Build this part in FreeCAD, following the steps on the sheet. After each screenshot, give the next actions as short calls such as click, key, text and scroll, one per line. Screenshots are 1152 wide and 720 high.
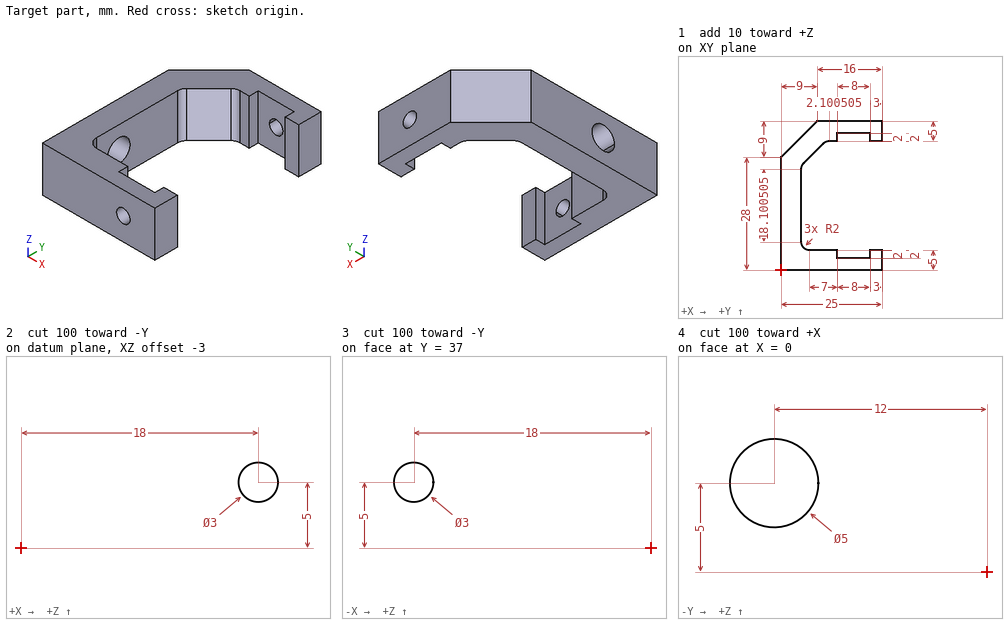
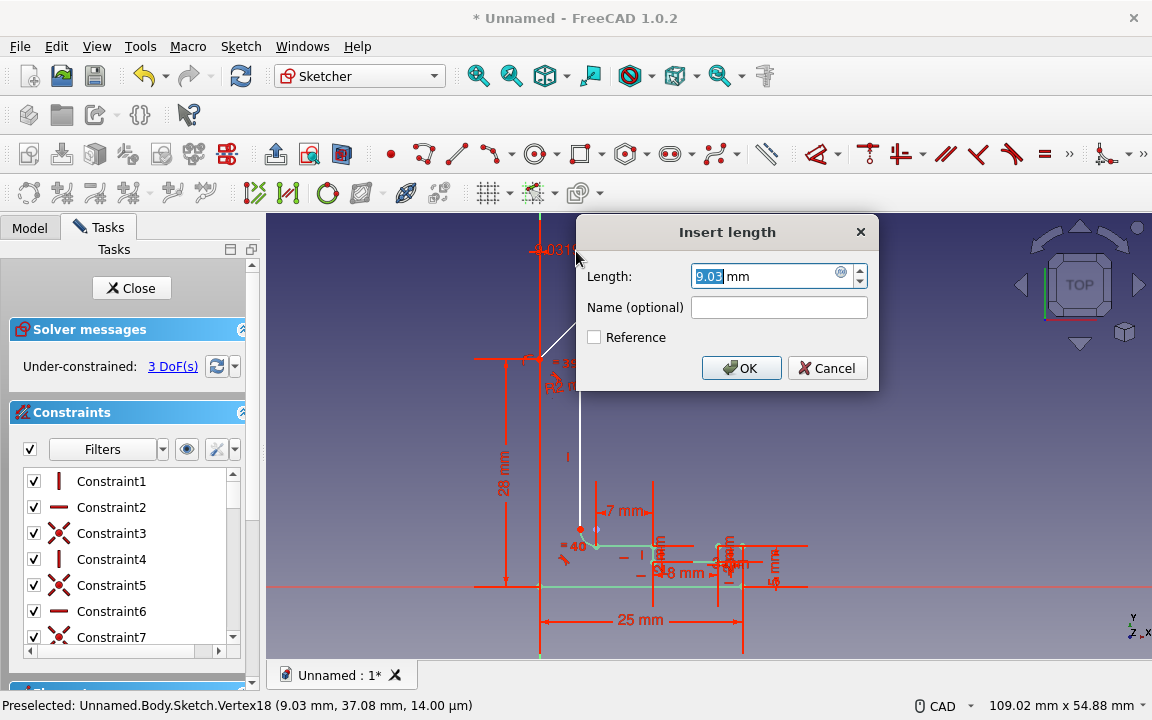
text(9)
key(Return)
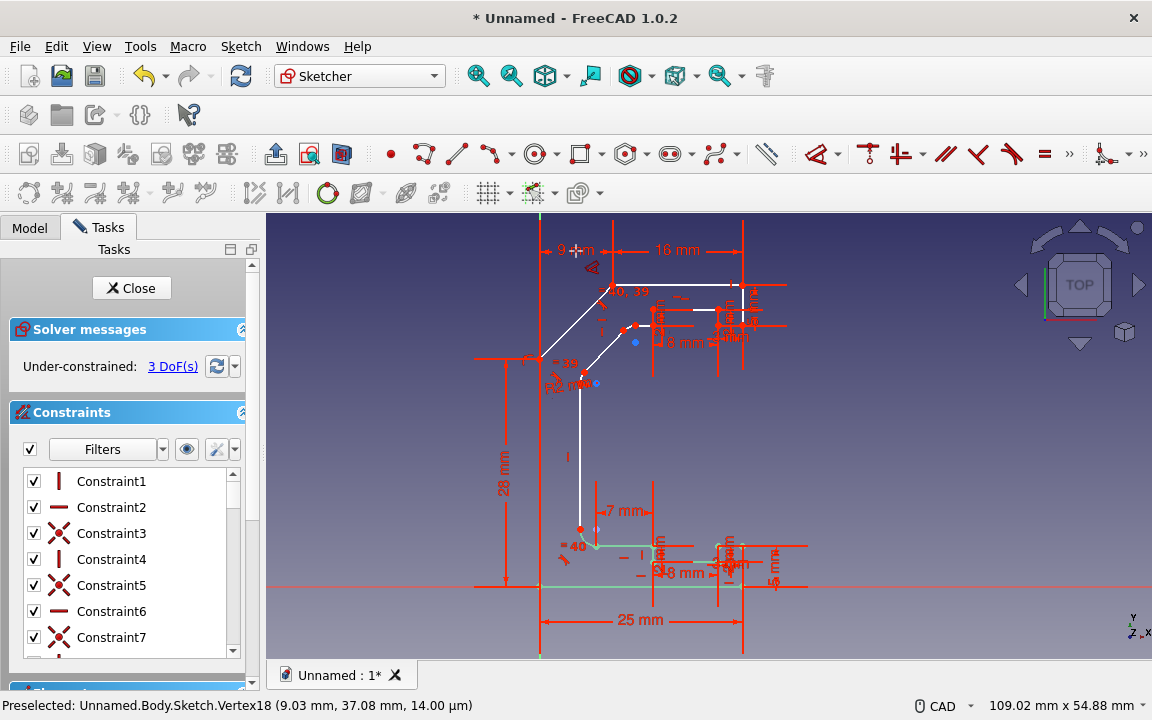
click(591, 307)
click(506, 322)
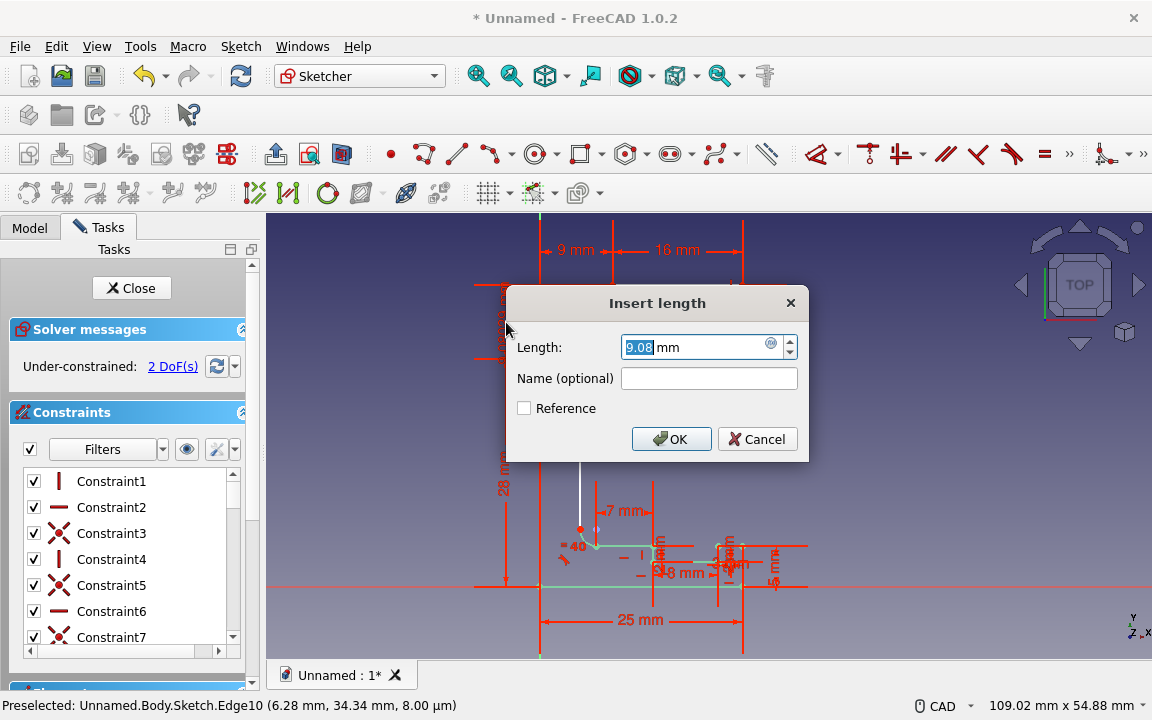
text(9)
key(Return)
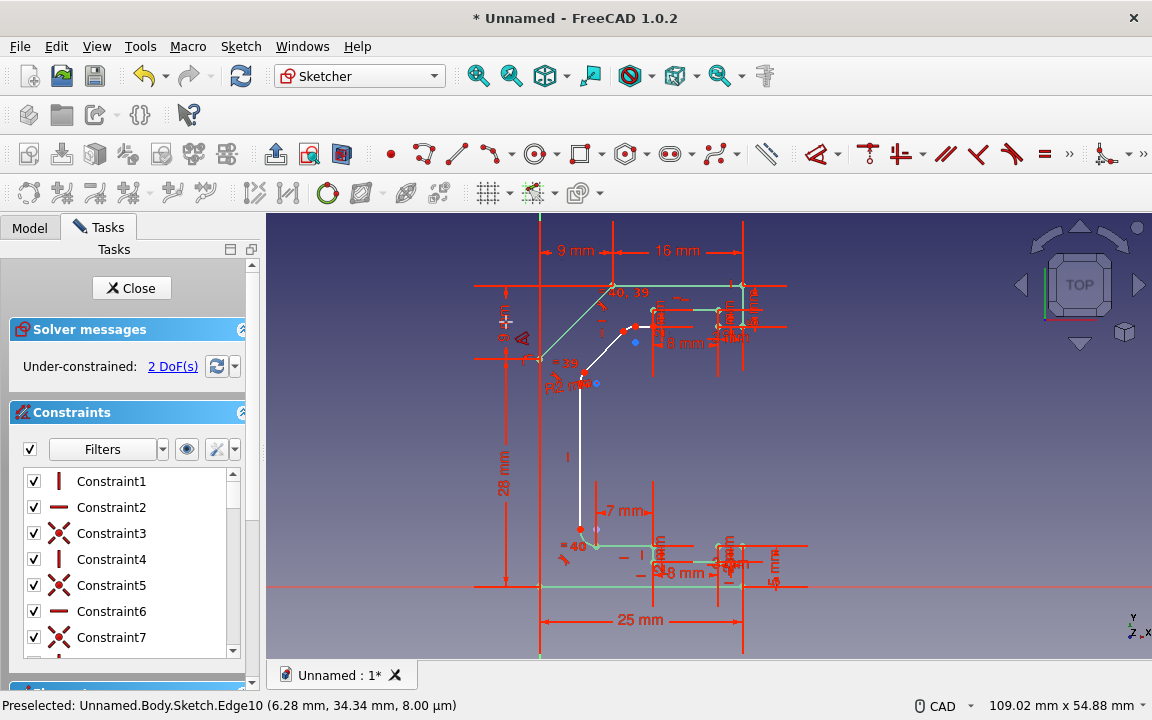
scroll(644, 327, up, 5)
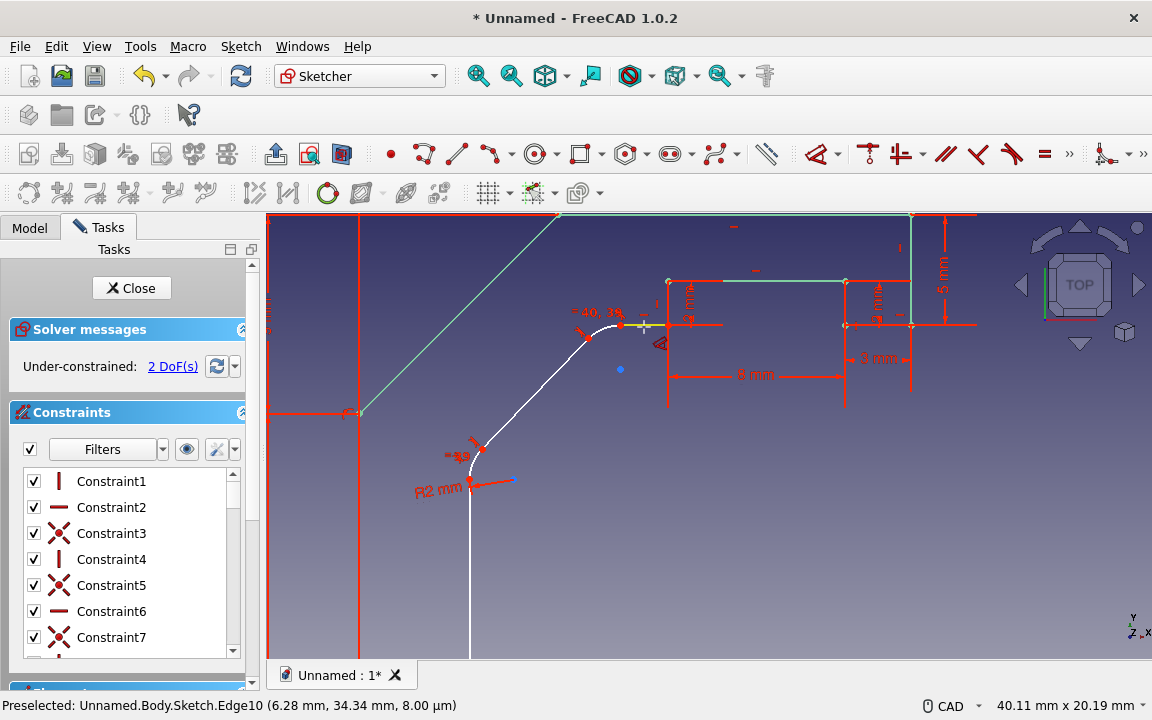
click(644, 325)
click(644, 359)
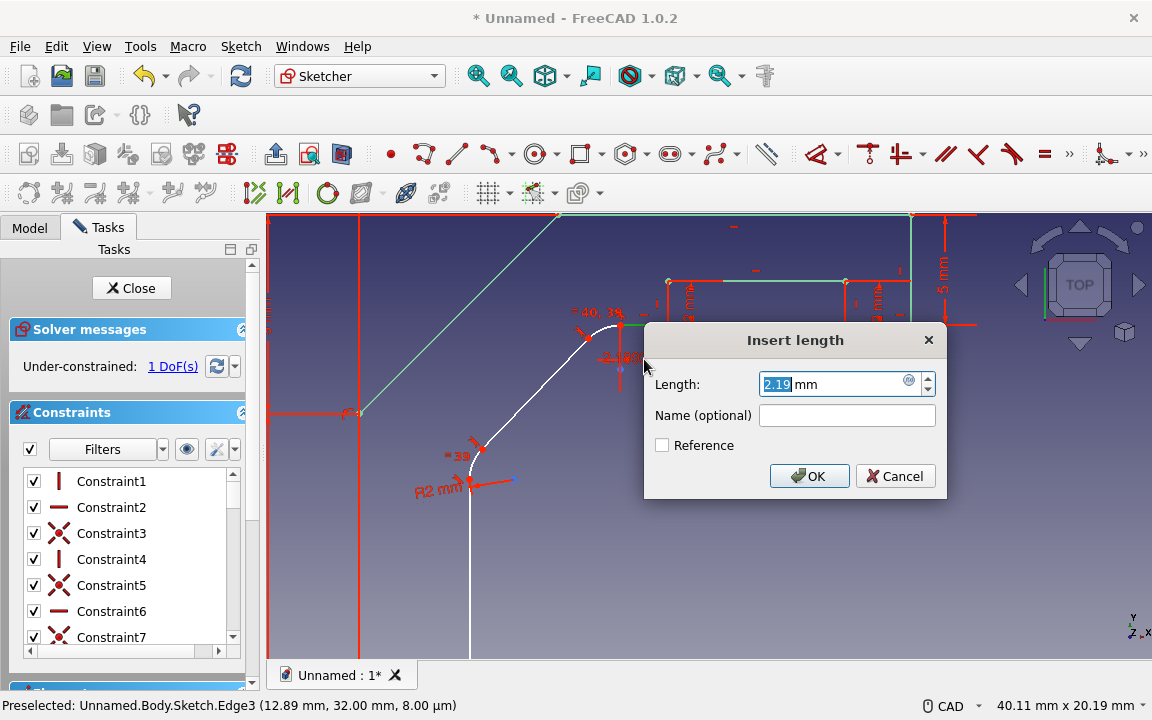
text(2.100505)
key(Return)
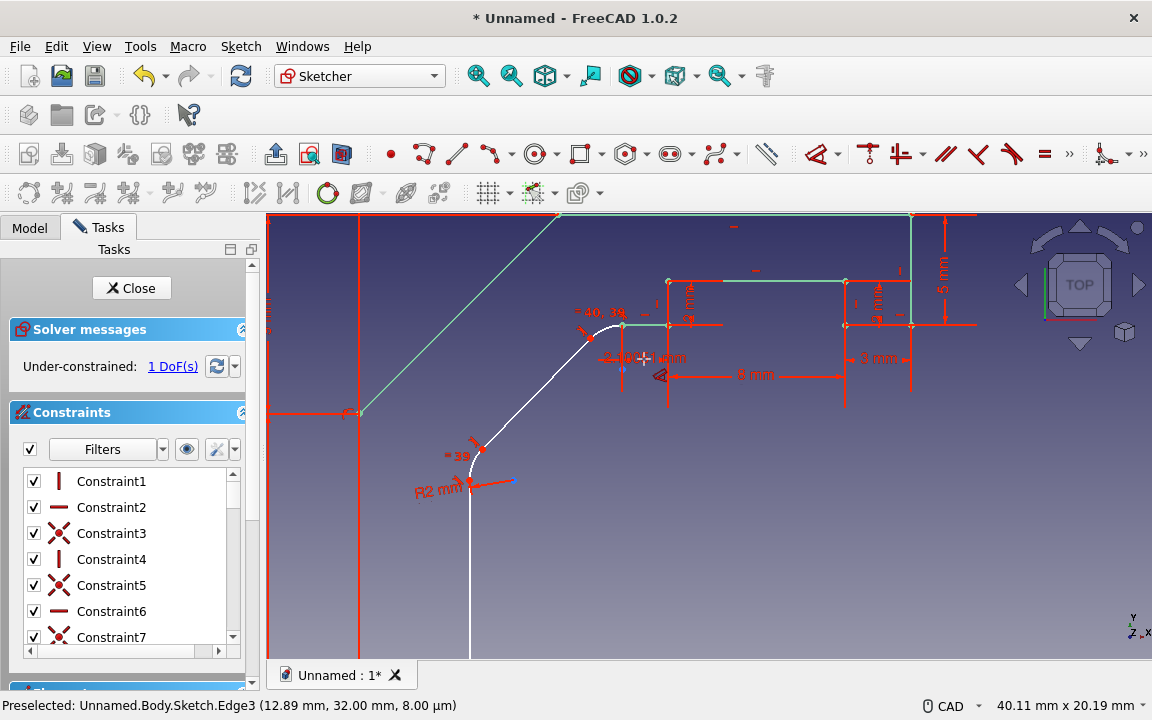
click(470, 599)
click(436, 556)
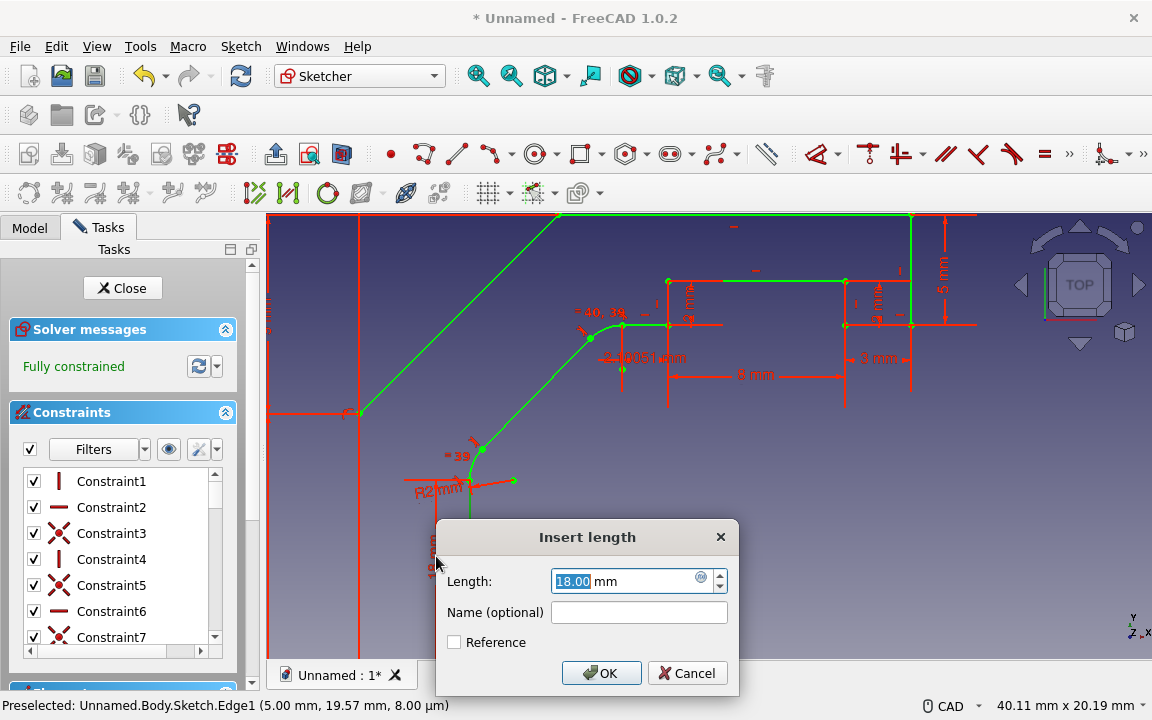
text(18.100505)
key(Return)
key(Escape)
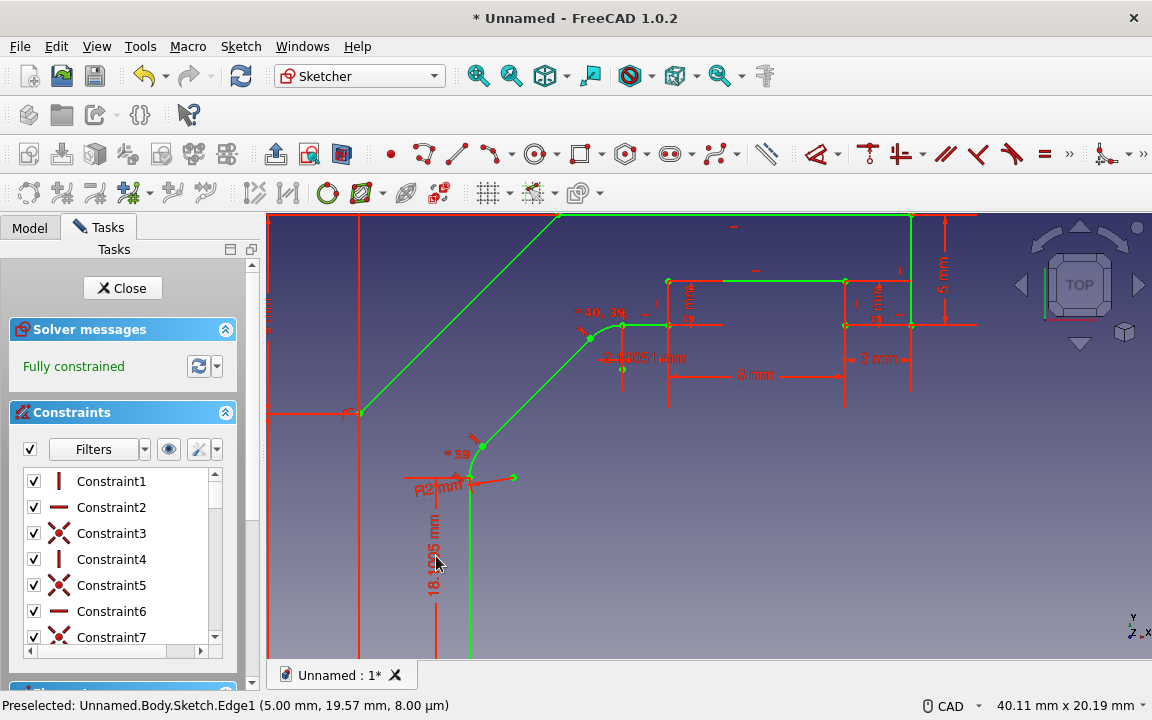
click(123, 288)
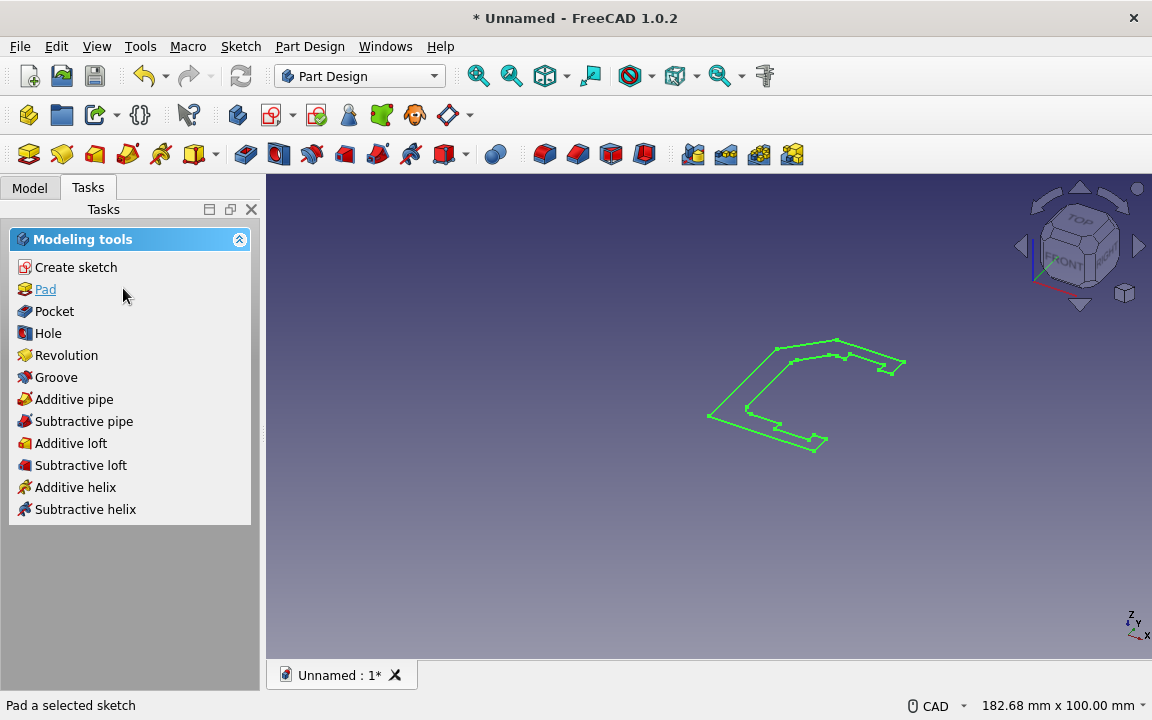
click(29, 154)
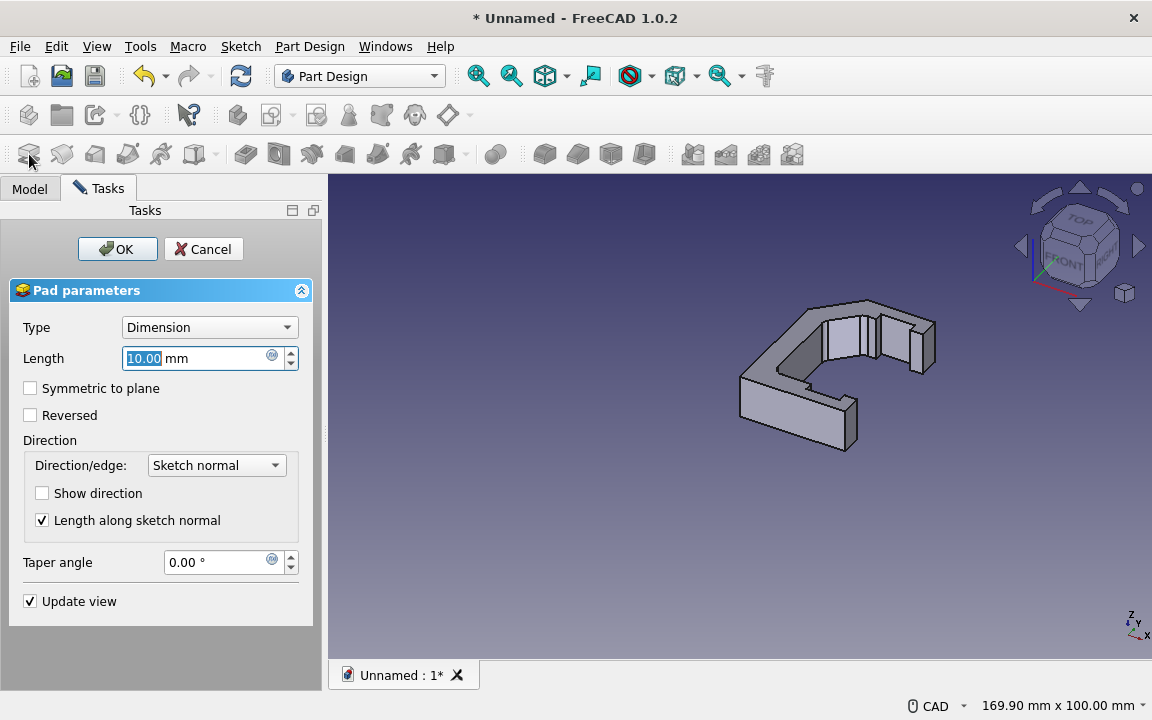
text(10)
key(Tab)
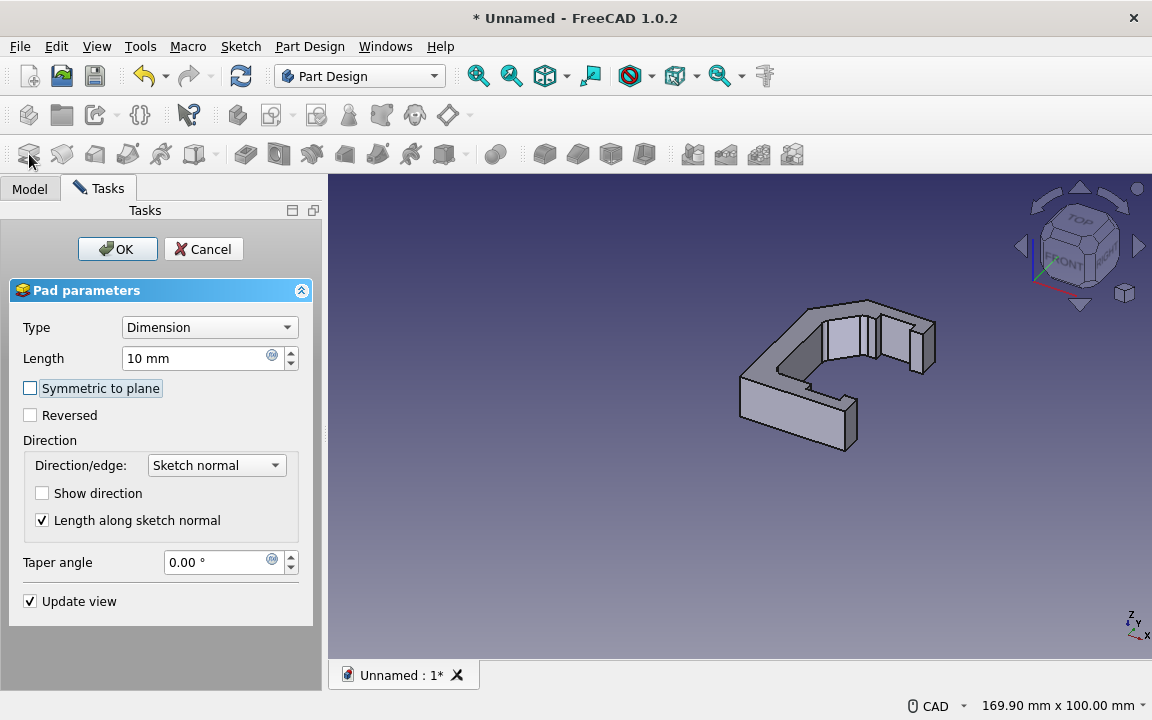
click(118, 249)